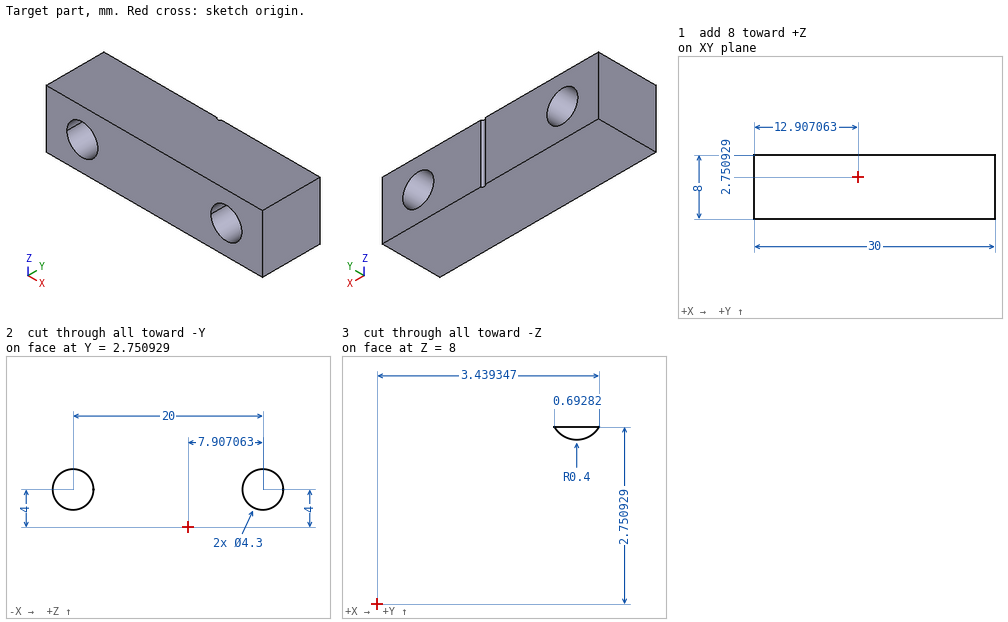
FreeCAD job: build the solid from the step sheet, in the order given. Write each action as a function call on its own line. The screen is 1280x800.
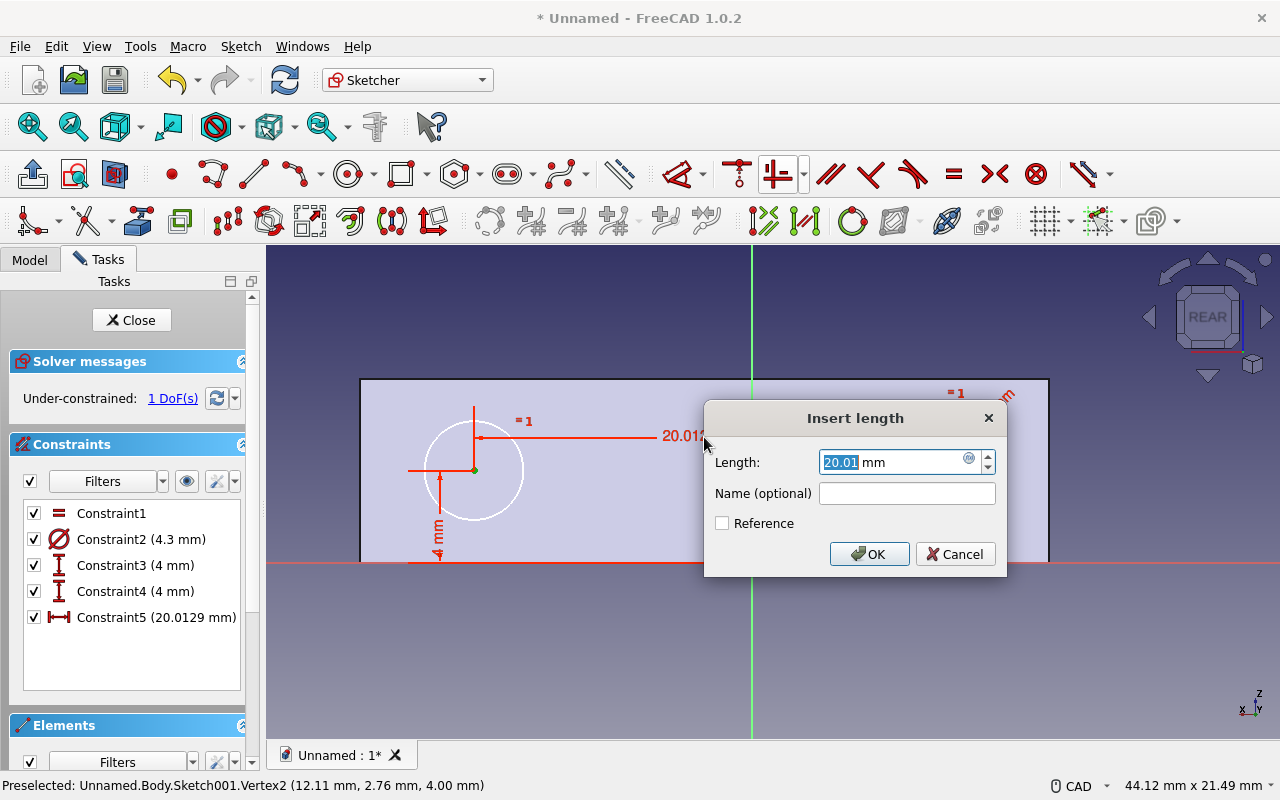
text(20)
key(Return)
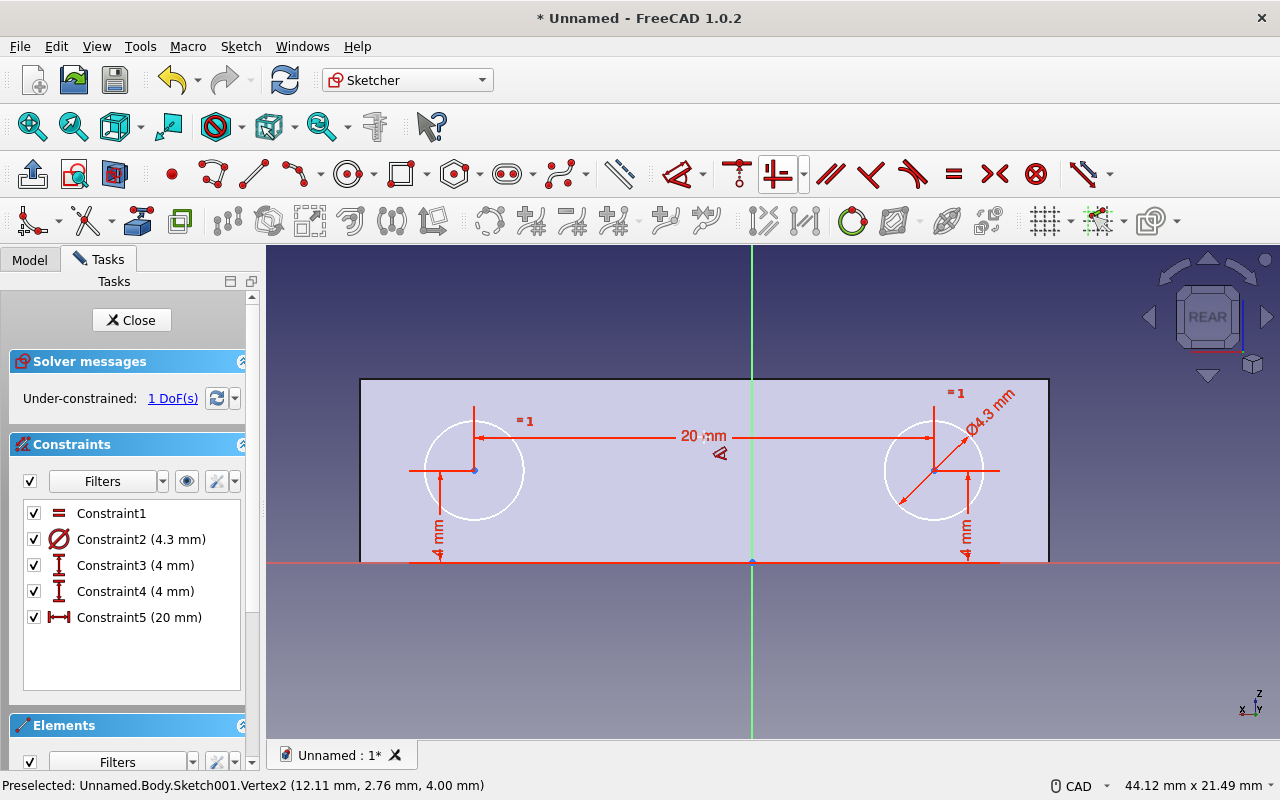
click(934, 471)
click(843, 597)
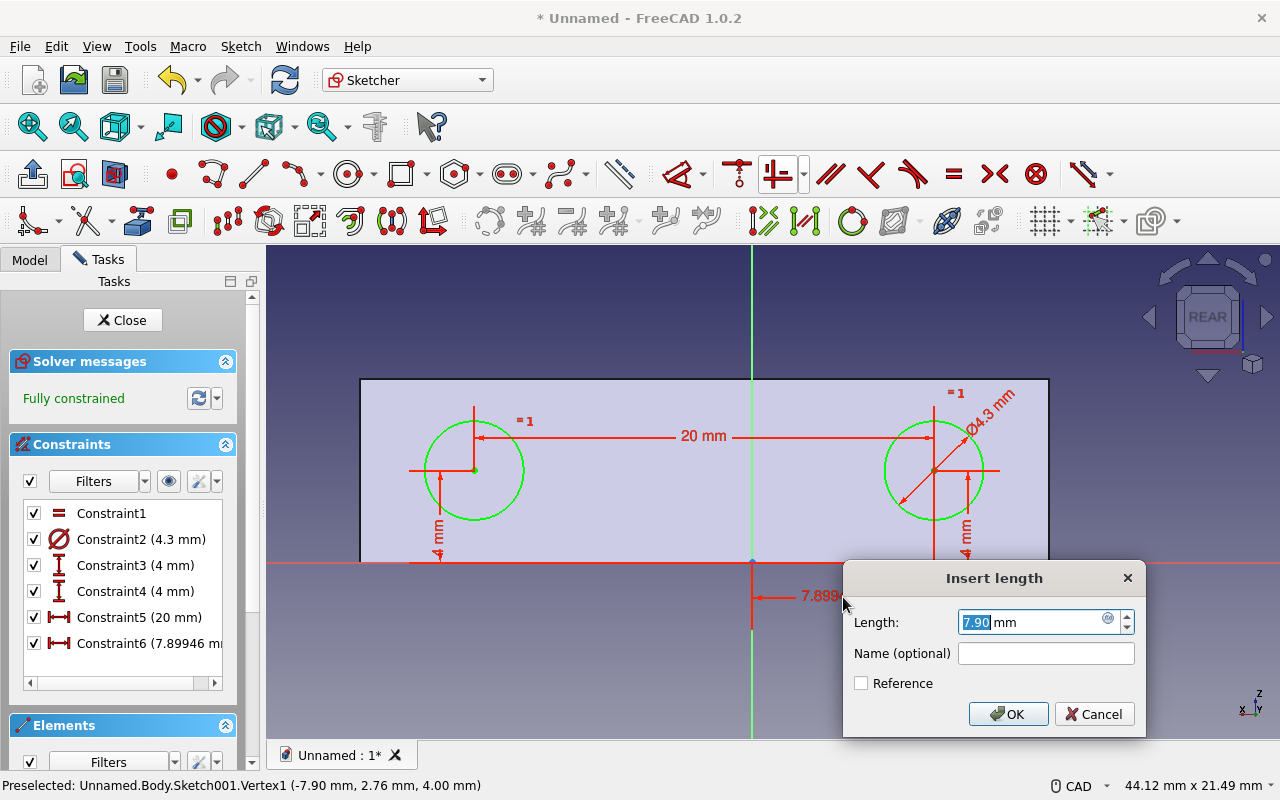
text(7.907063)
key(Return)
key(Escape)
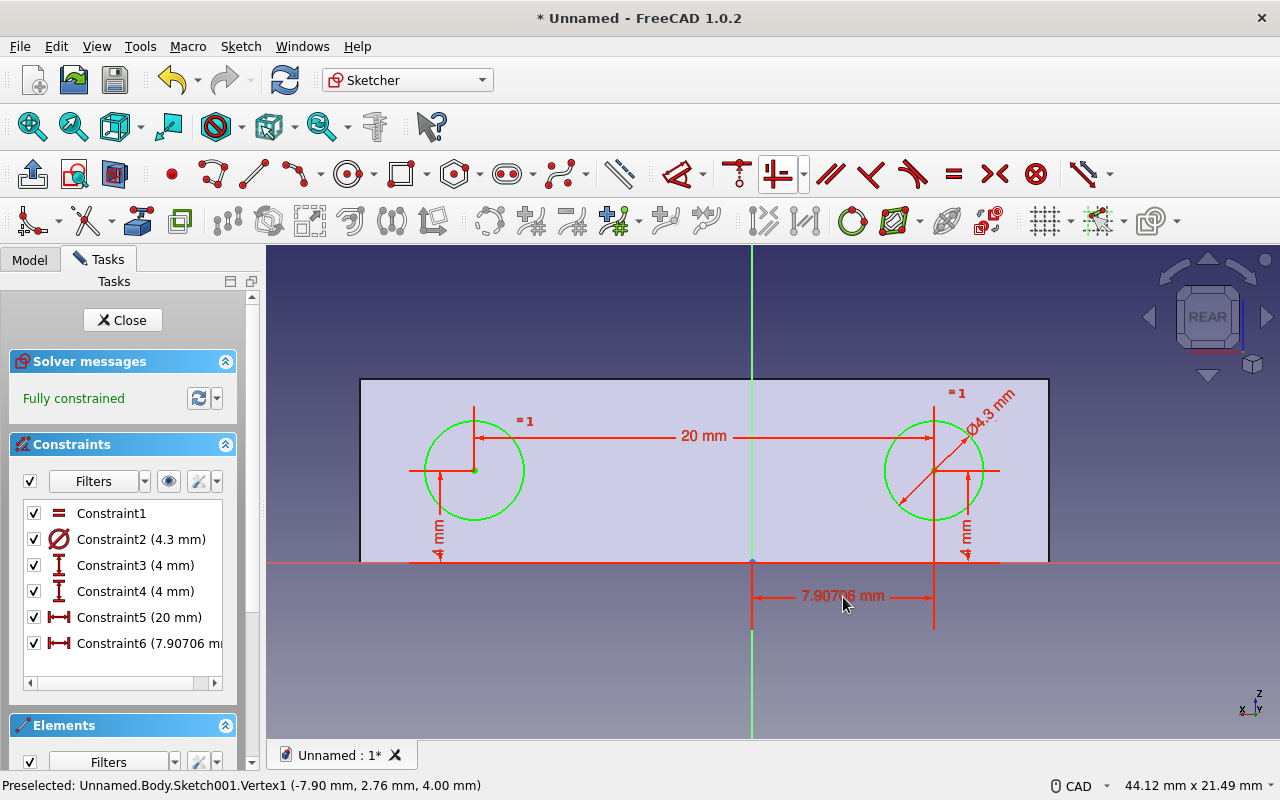
click(123, 320)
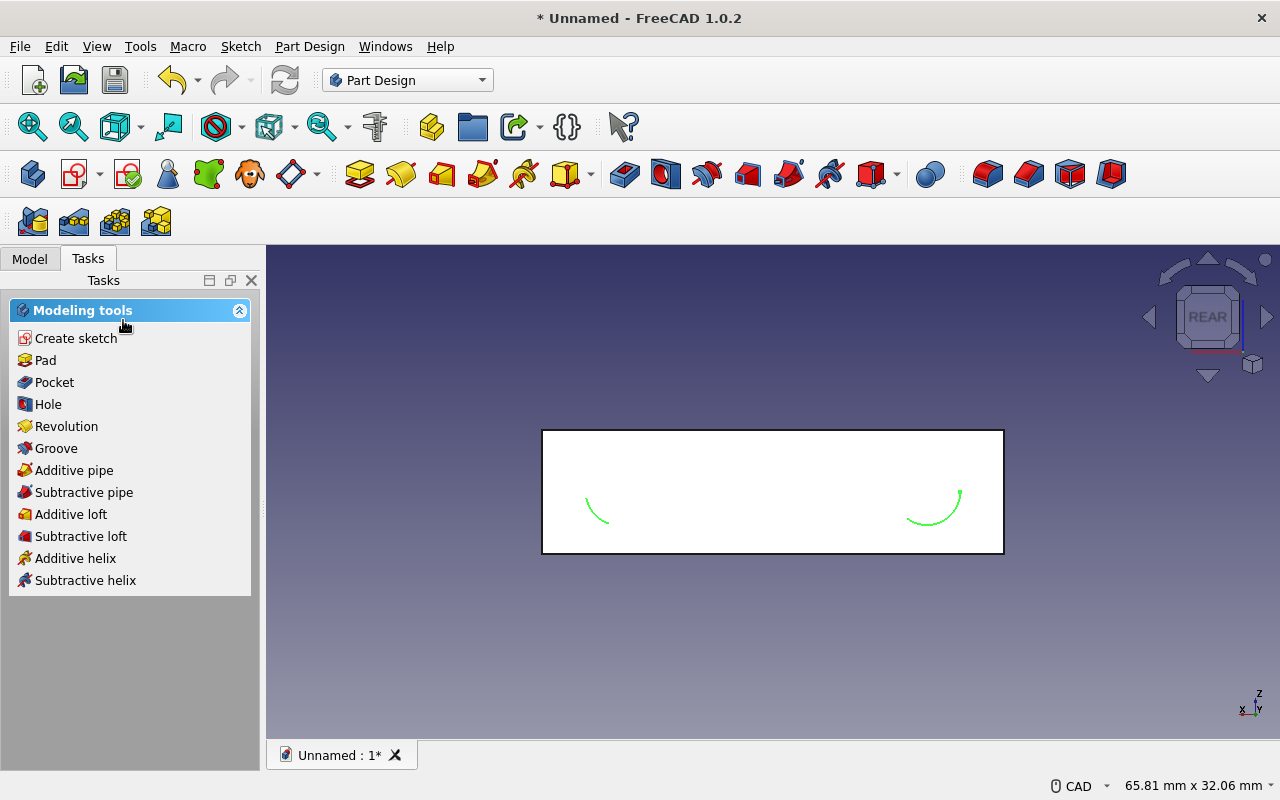
click(625, 174)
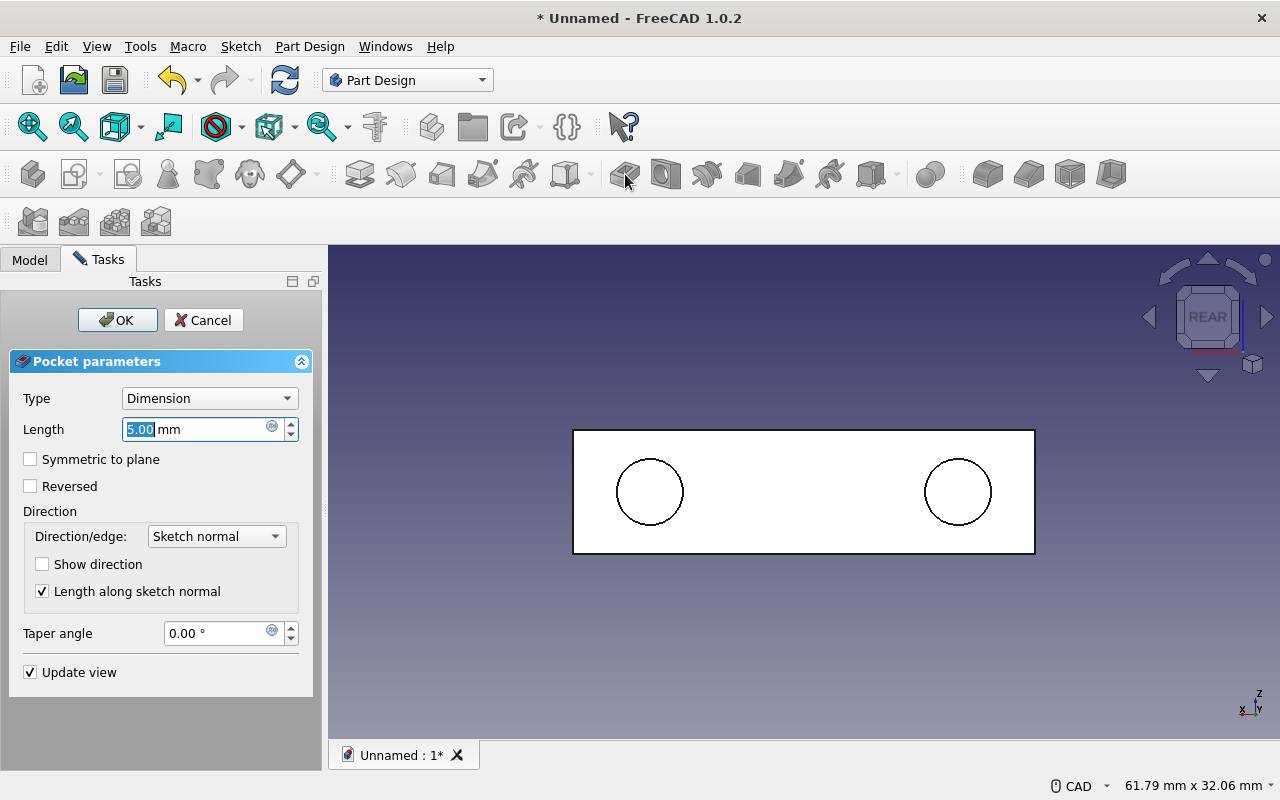
click(210, 398)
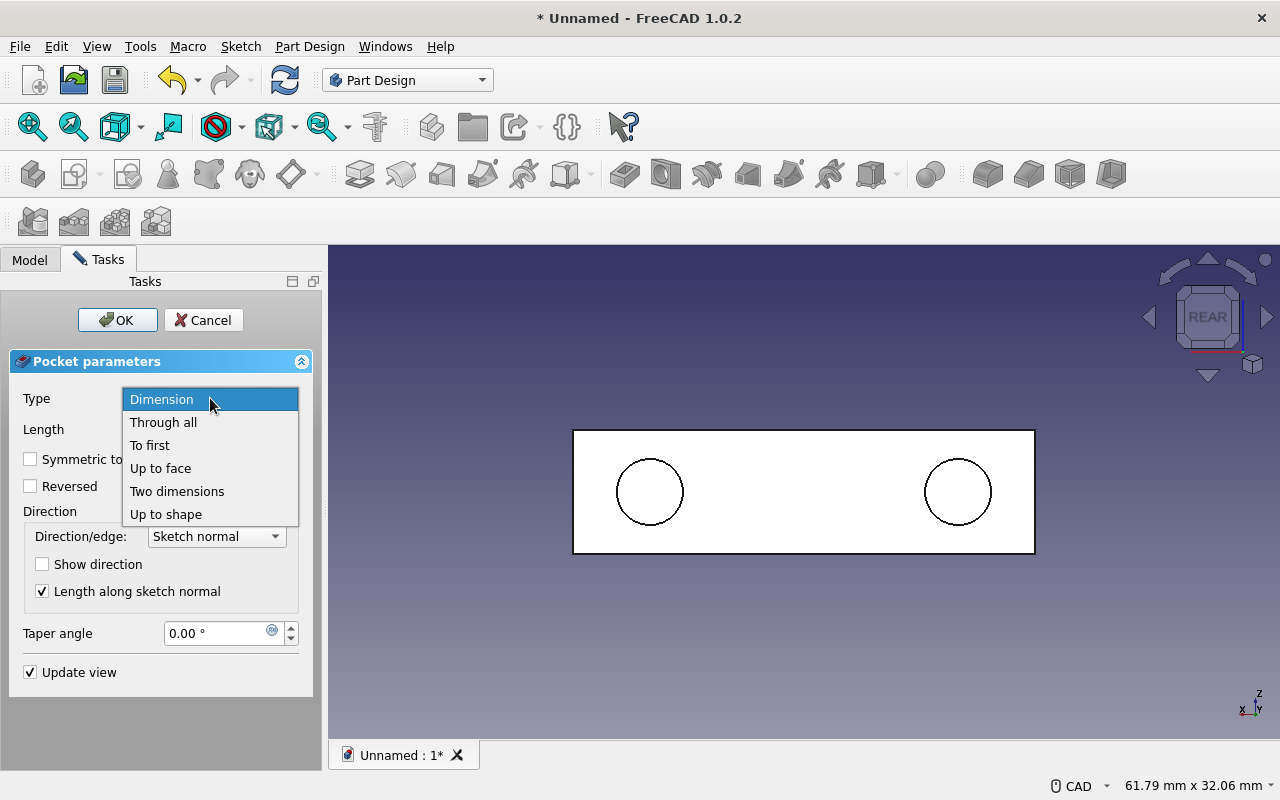
click(208, 422)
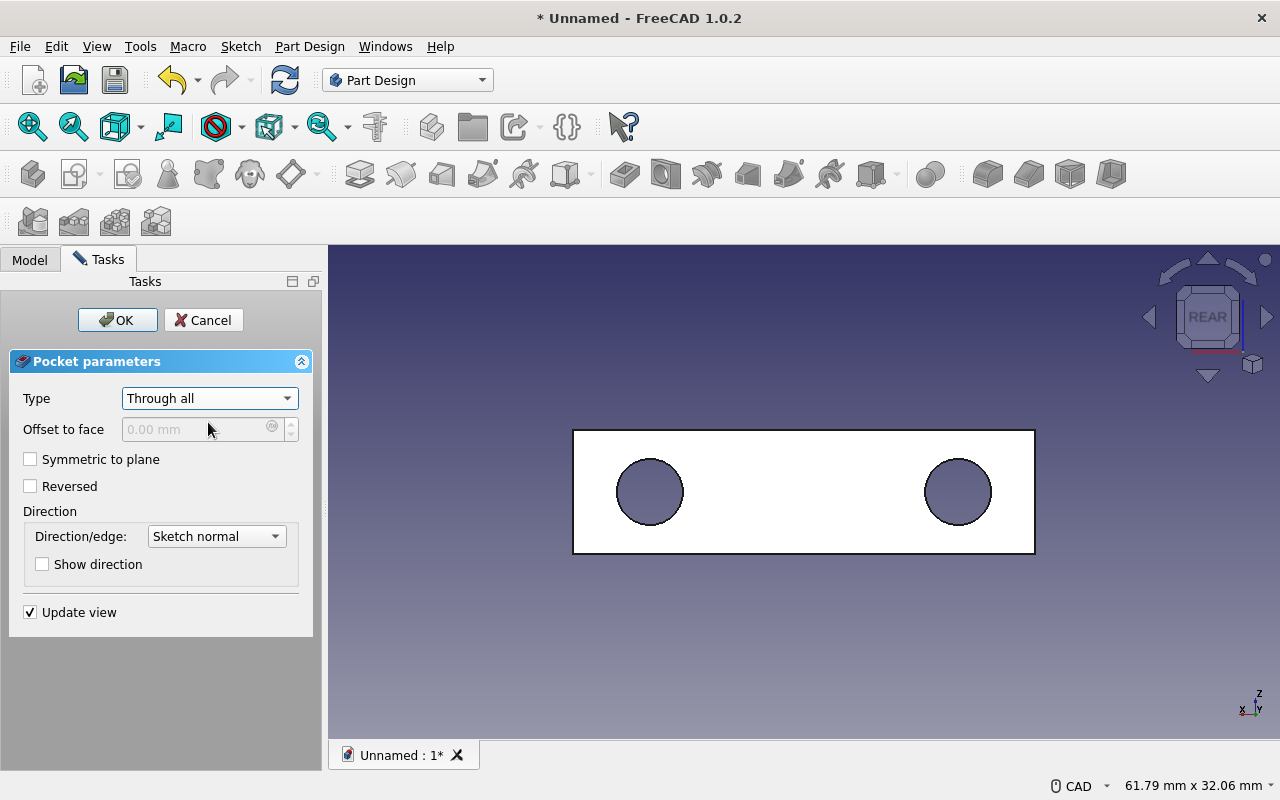
click(118, 320)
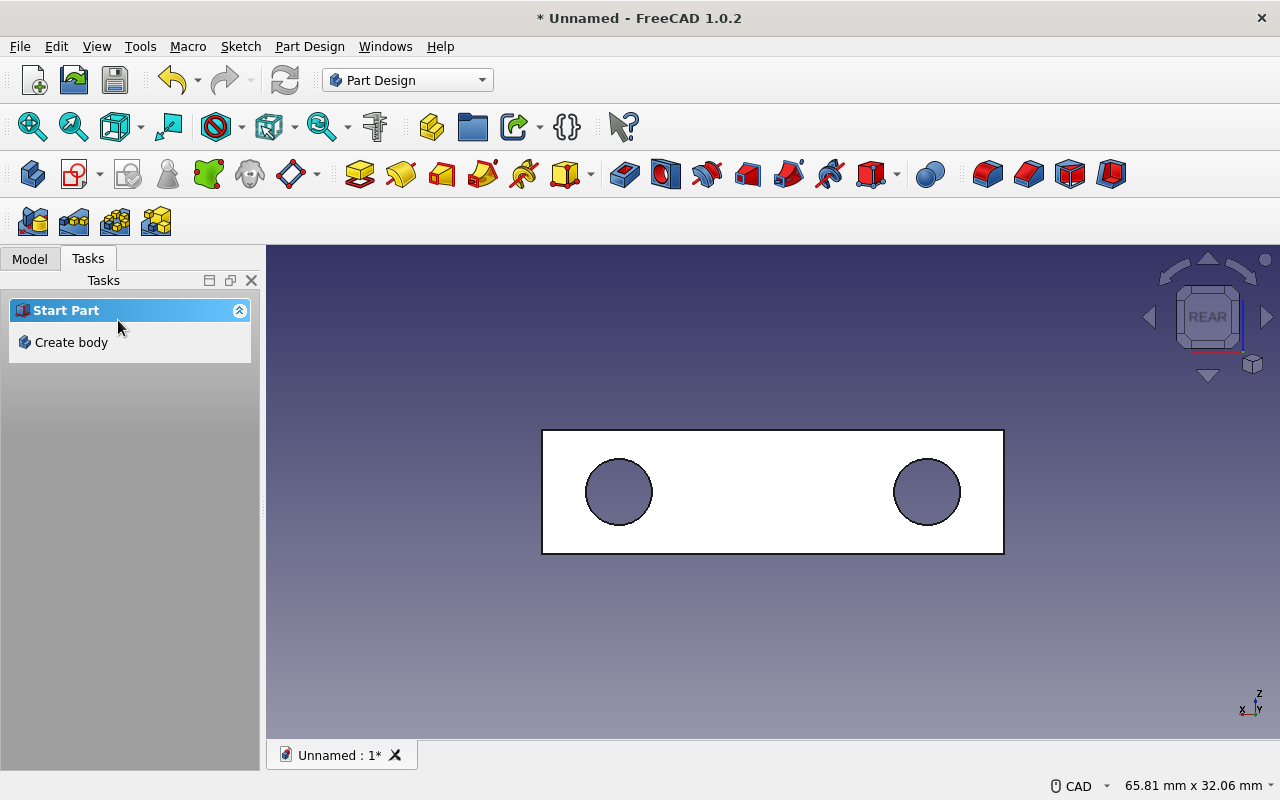
key(0)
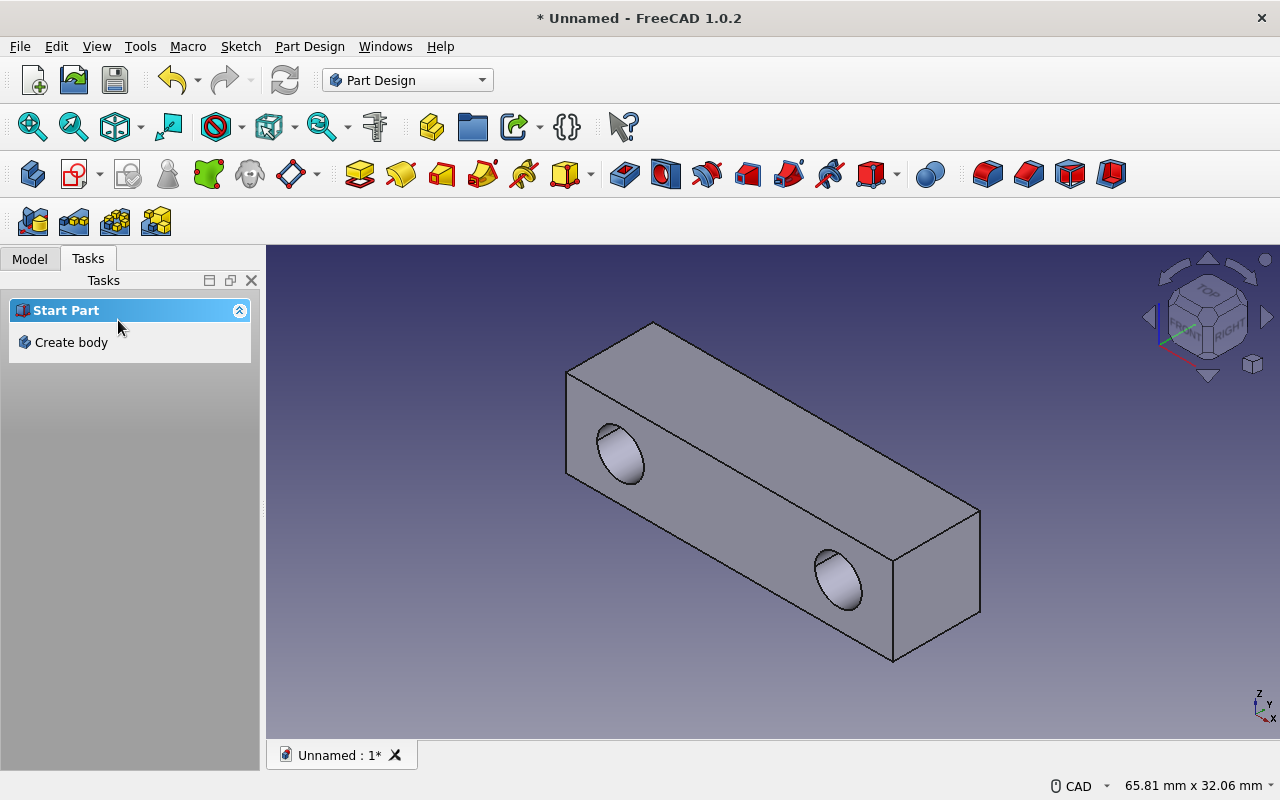
click(866, 495)